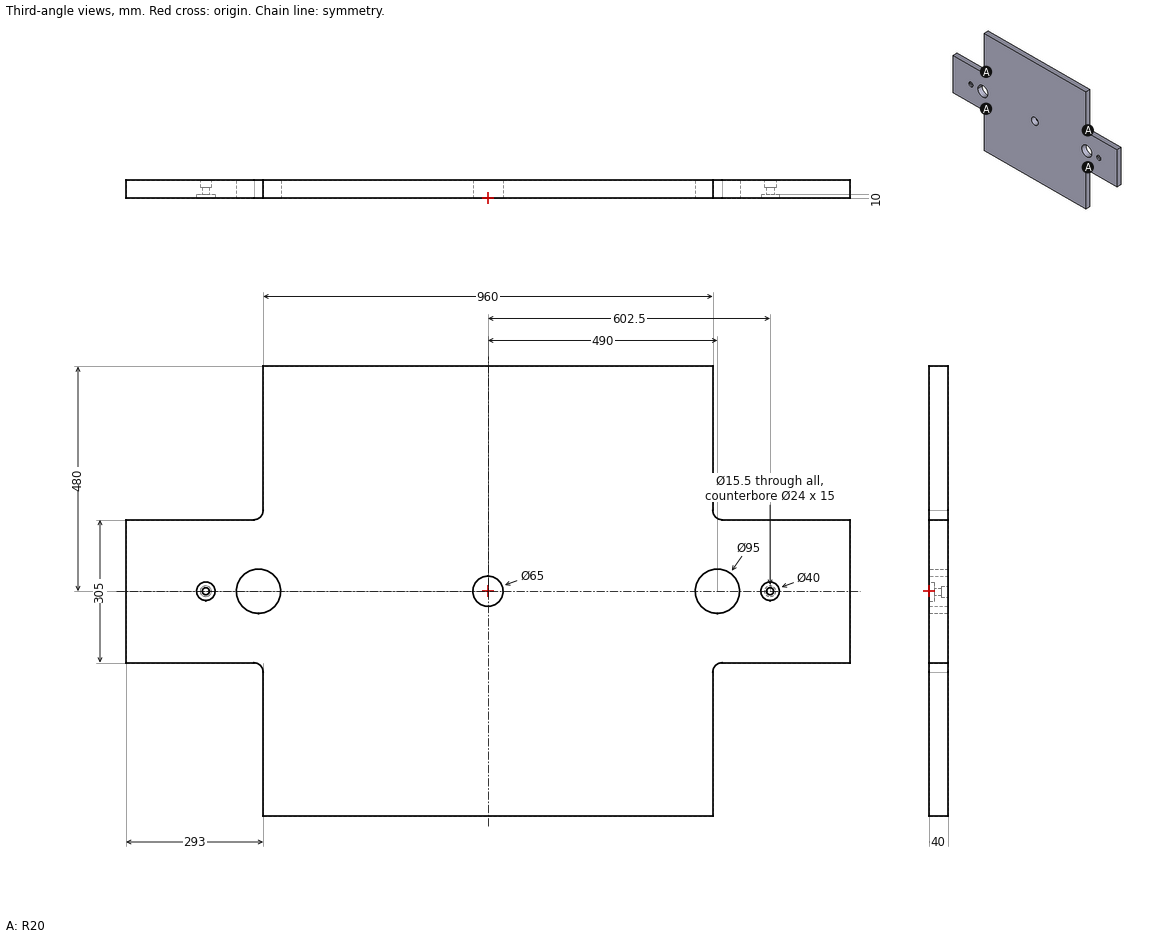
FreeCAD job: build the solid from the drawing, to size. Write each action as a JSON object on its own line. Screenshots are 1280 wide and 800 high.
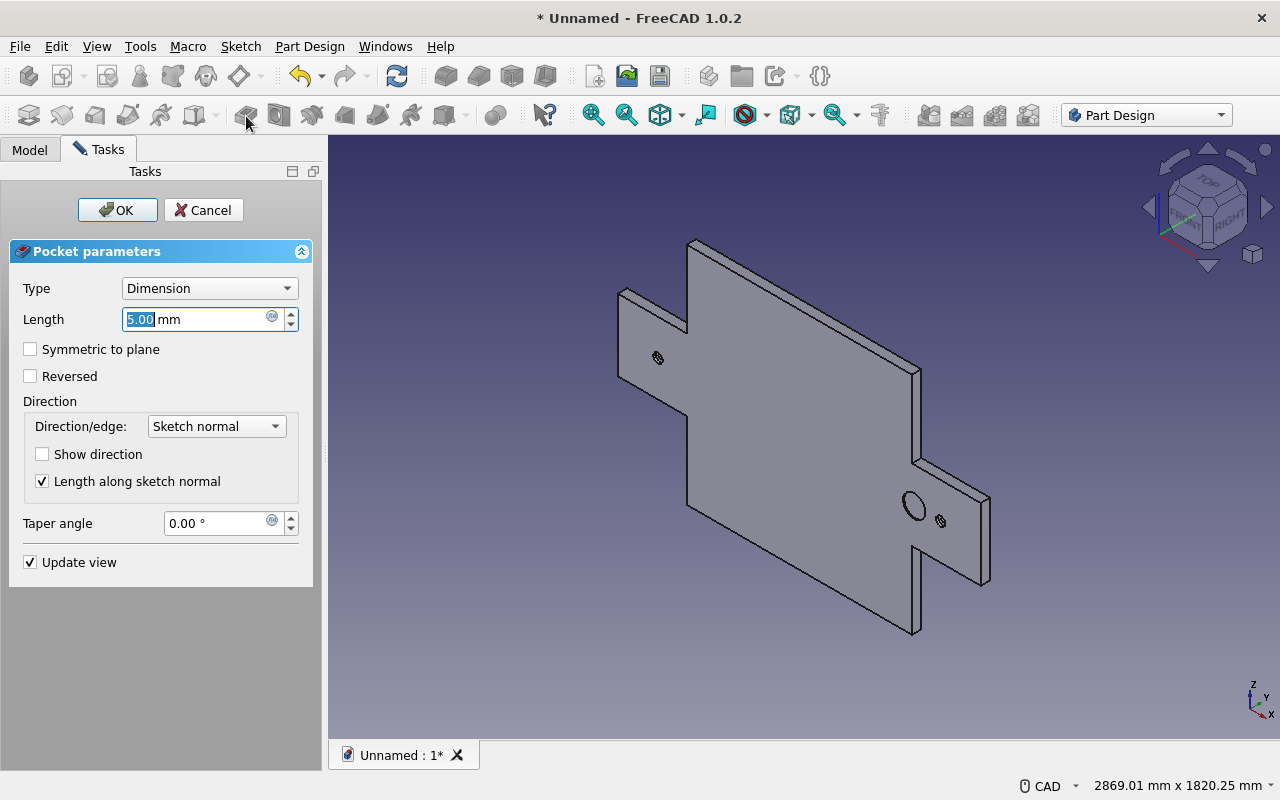
{"action": "left_click", "coordinate": [210, 288]}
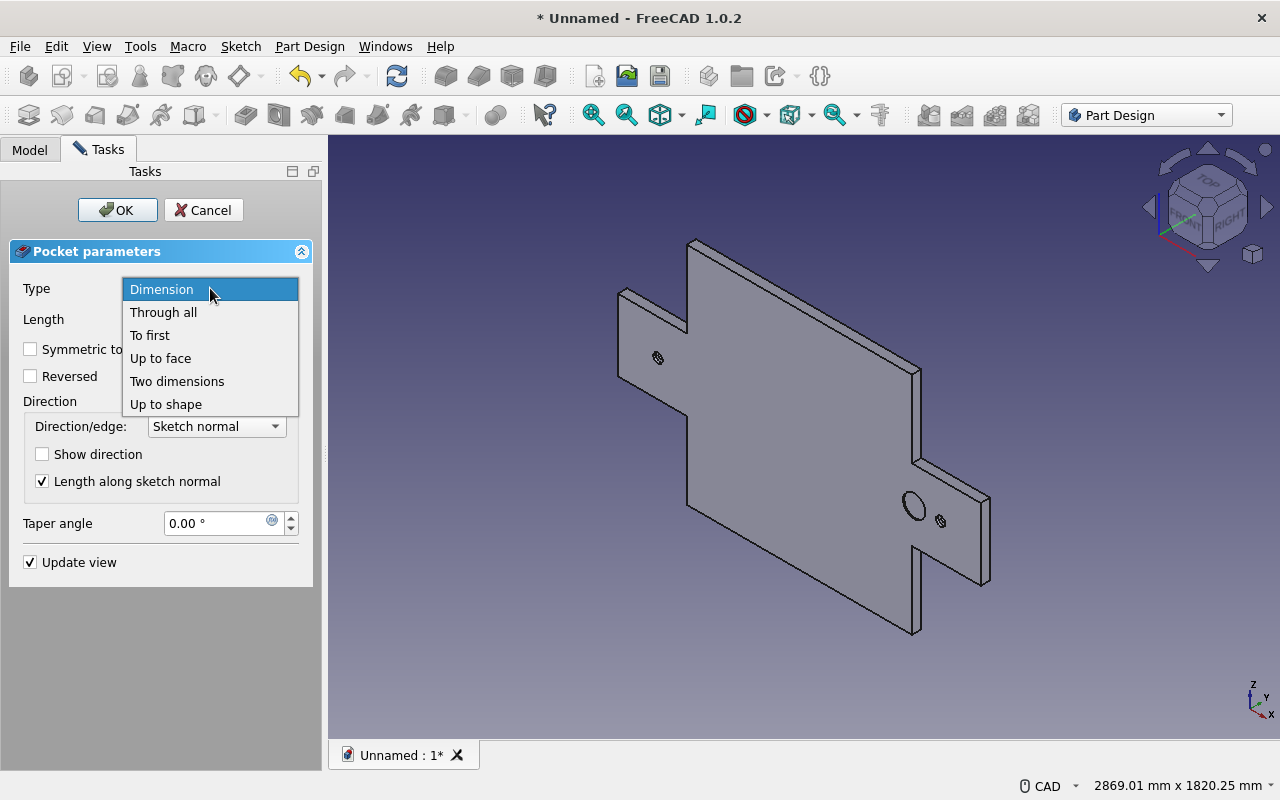
{"action": "left_click", "coordinate": [208, 312]}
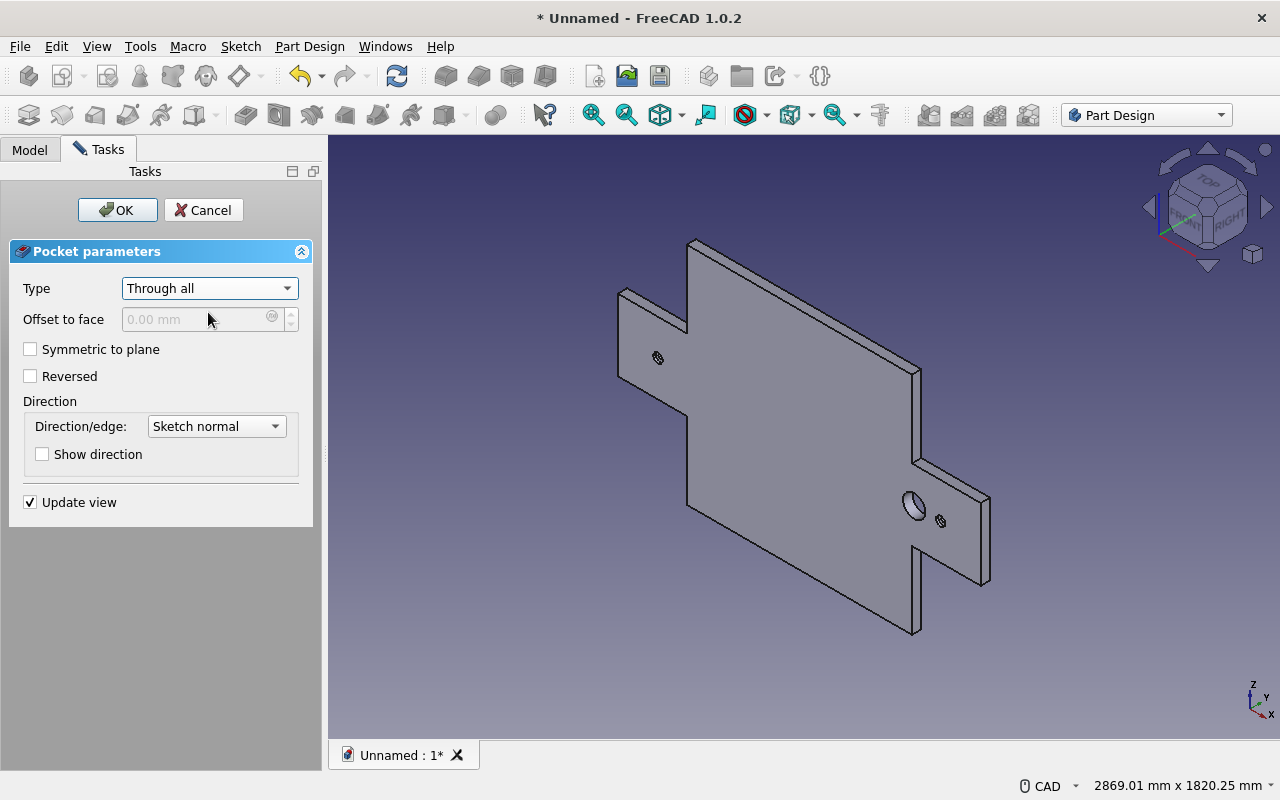
{"action": "left_click", "coordinate": [118, 210]}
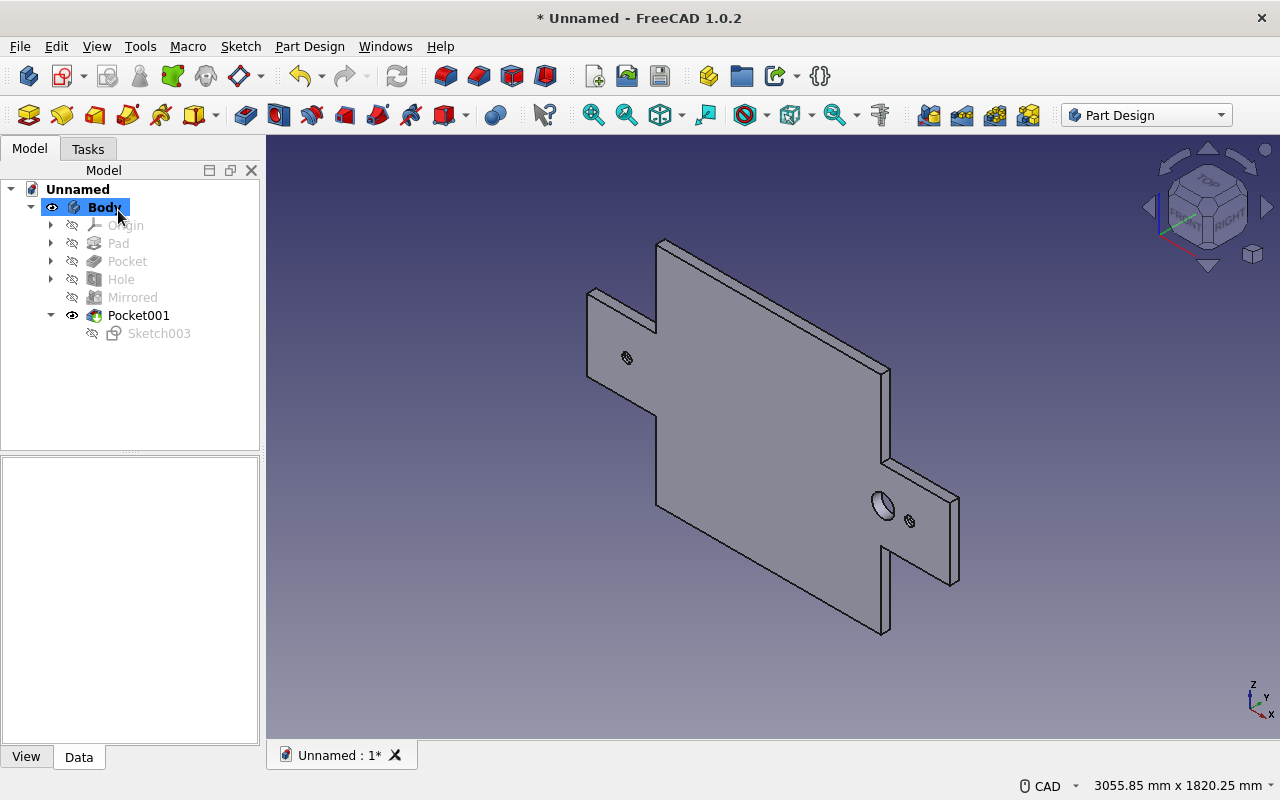
{"action": "left_click", "coordinate": [117, 315]}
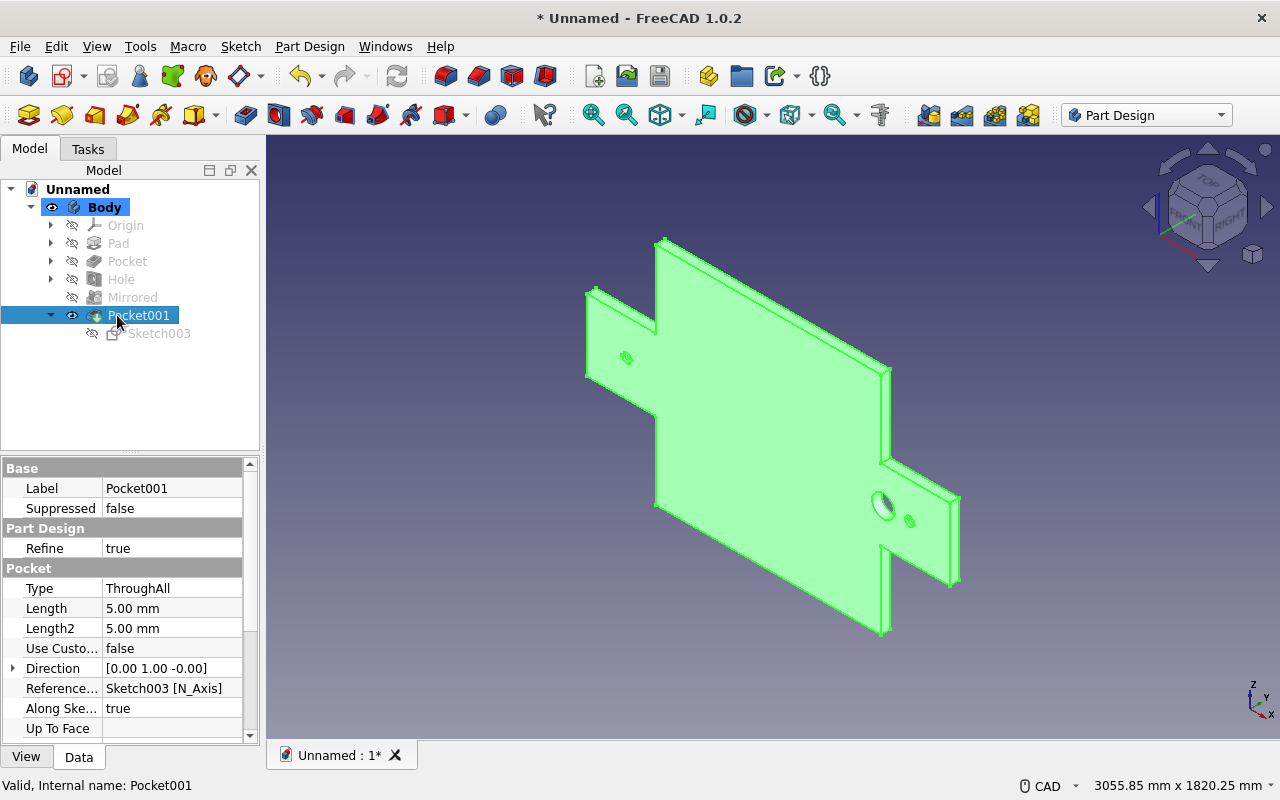
{"action": "left_click", "coordinate": [929, 116]}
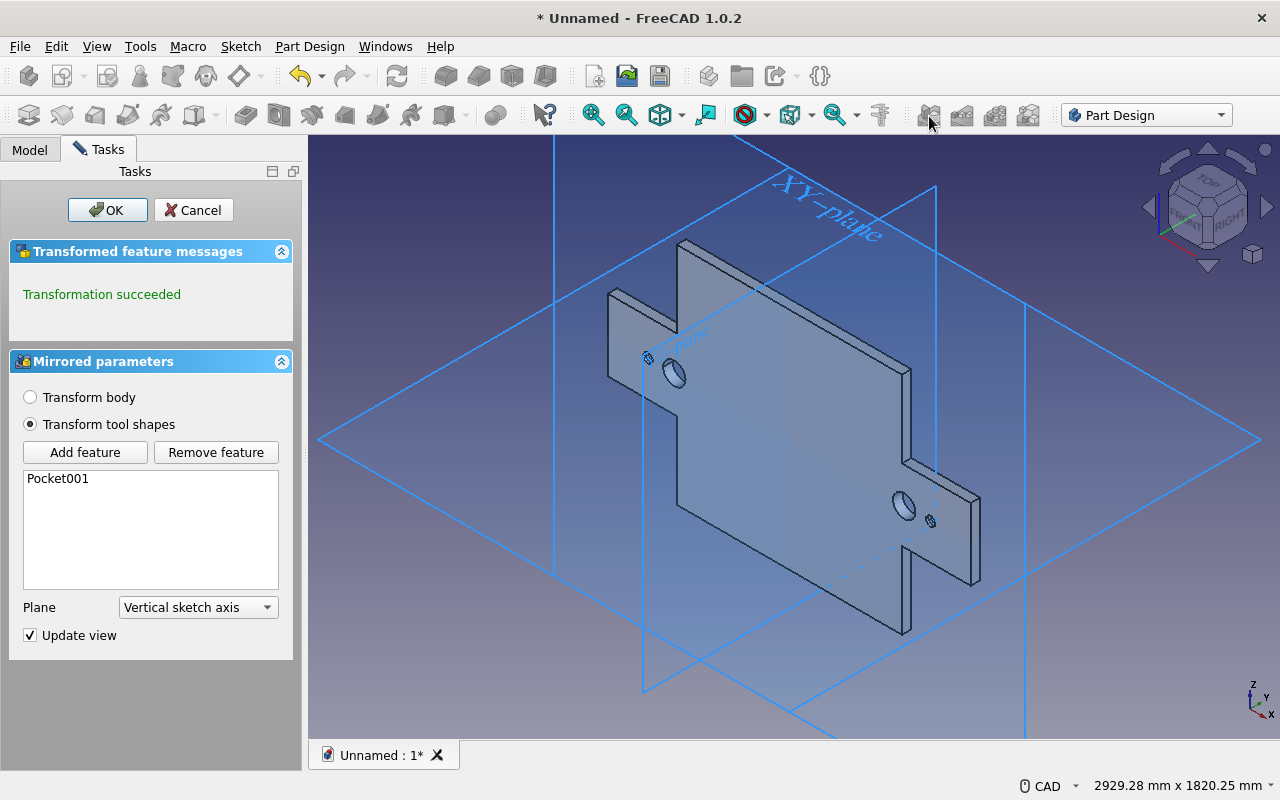
{"action": "left_click", "coordinate": [199, 608]}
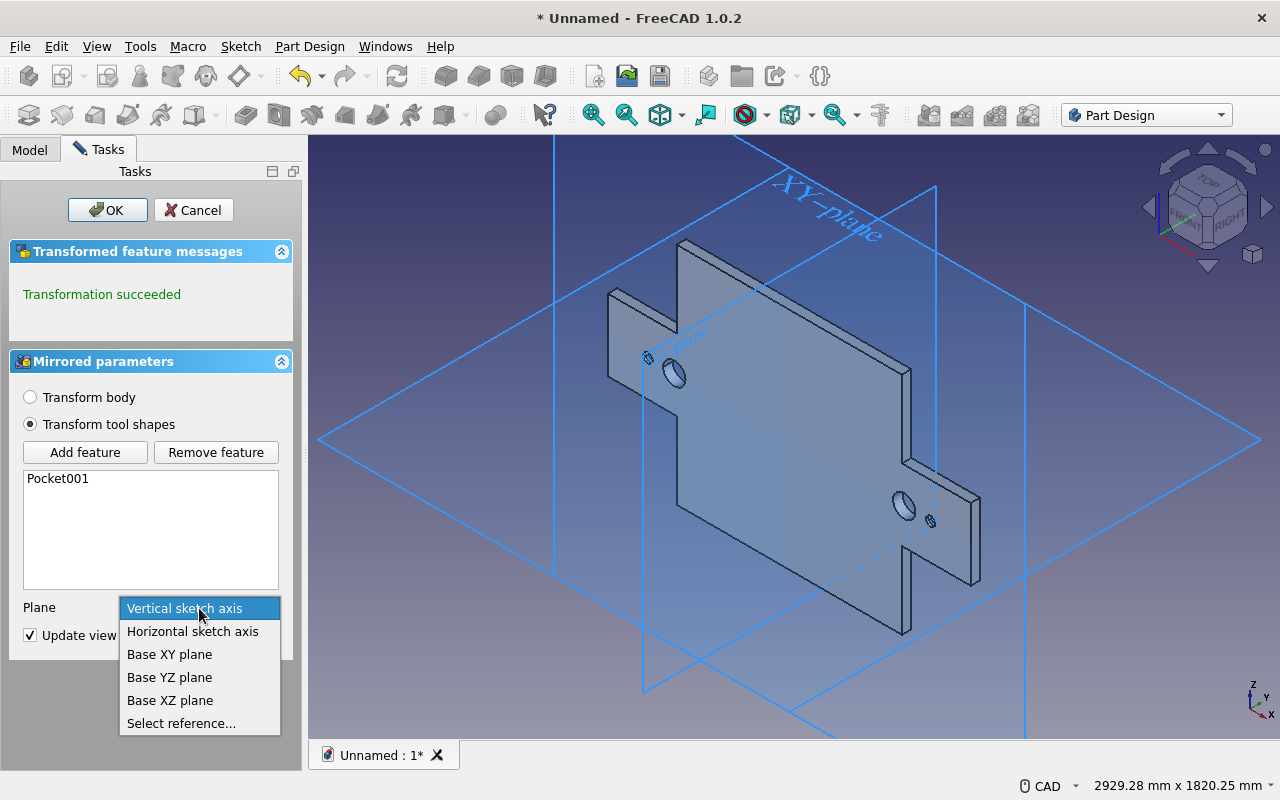
{"action": "left_click", "coordinate": [198, 678]}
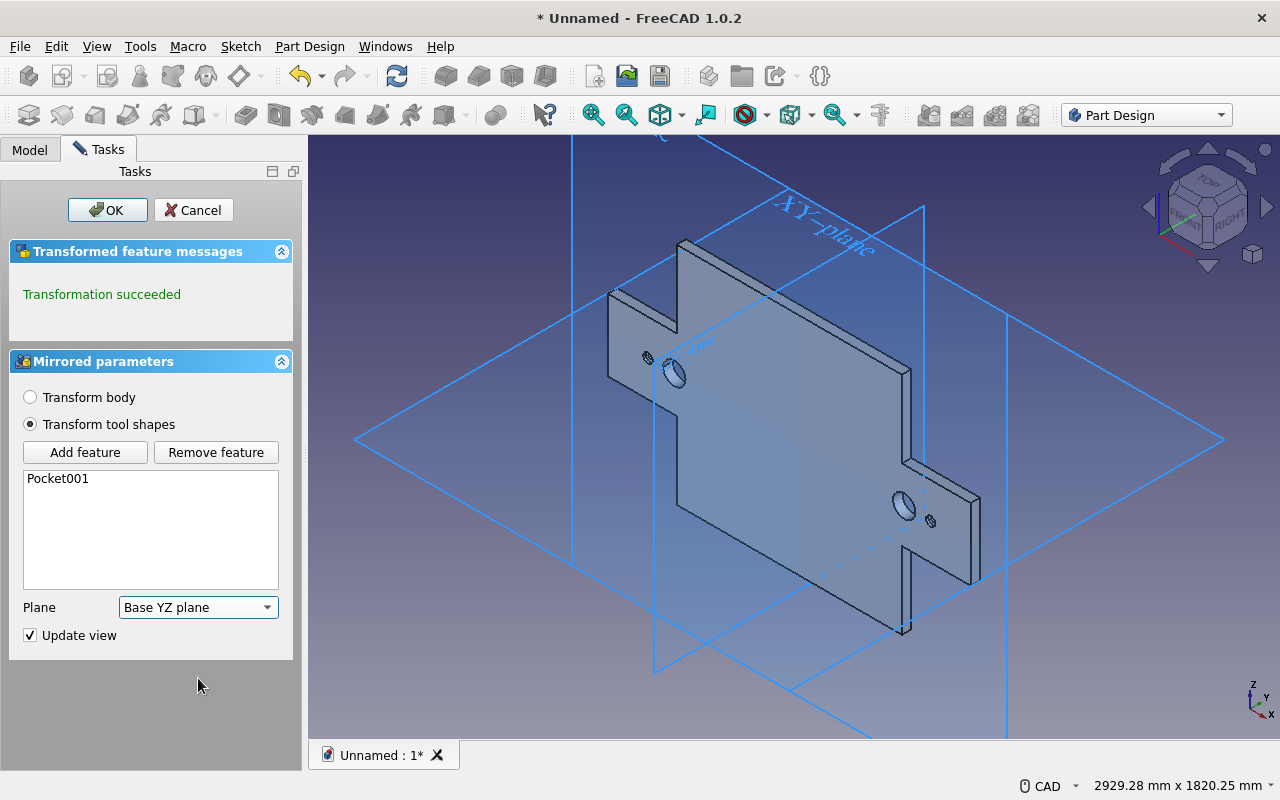
{"action": "left_click", "coordinate": [108, 210]}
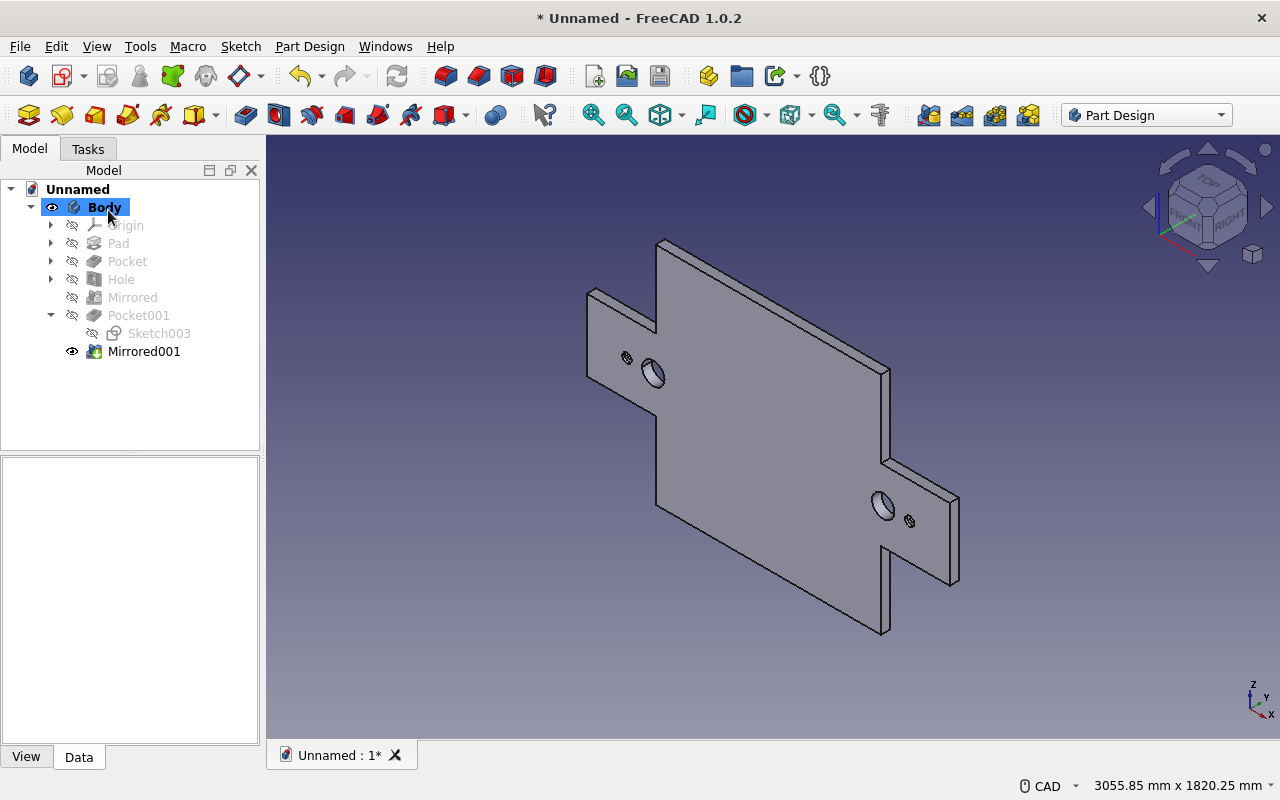
{"action": "key", "text": "4"}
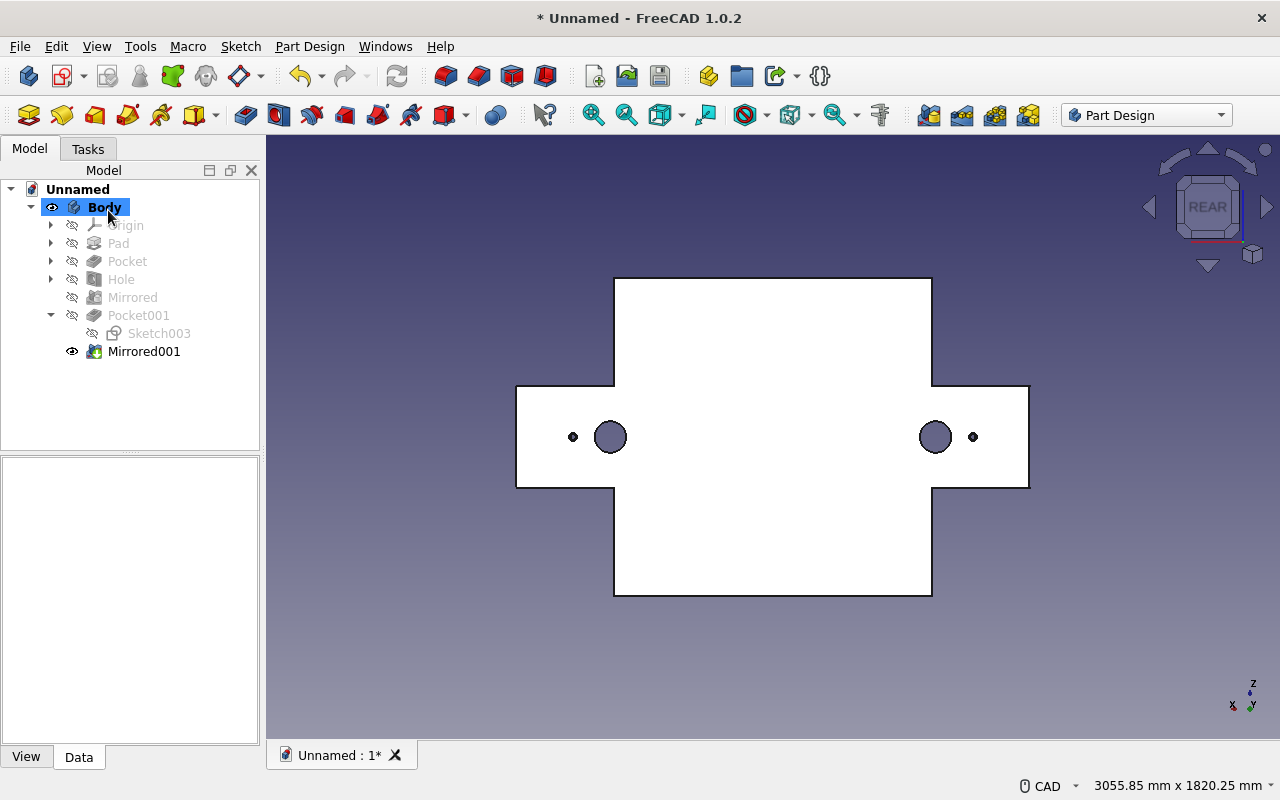
{"action": "left_click", "coordinate": [773, 436]}